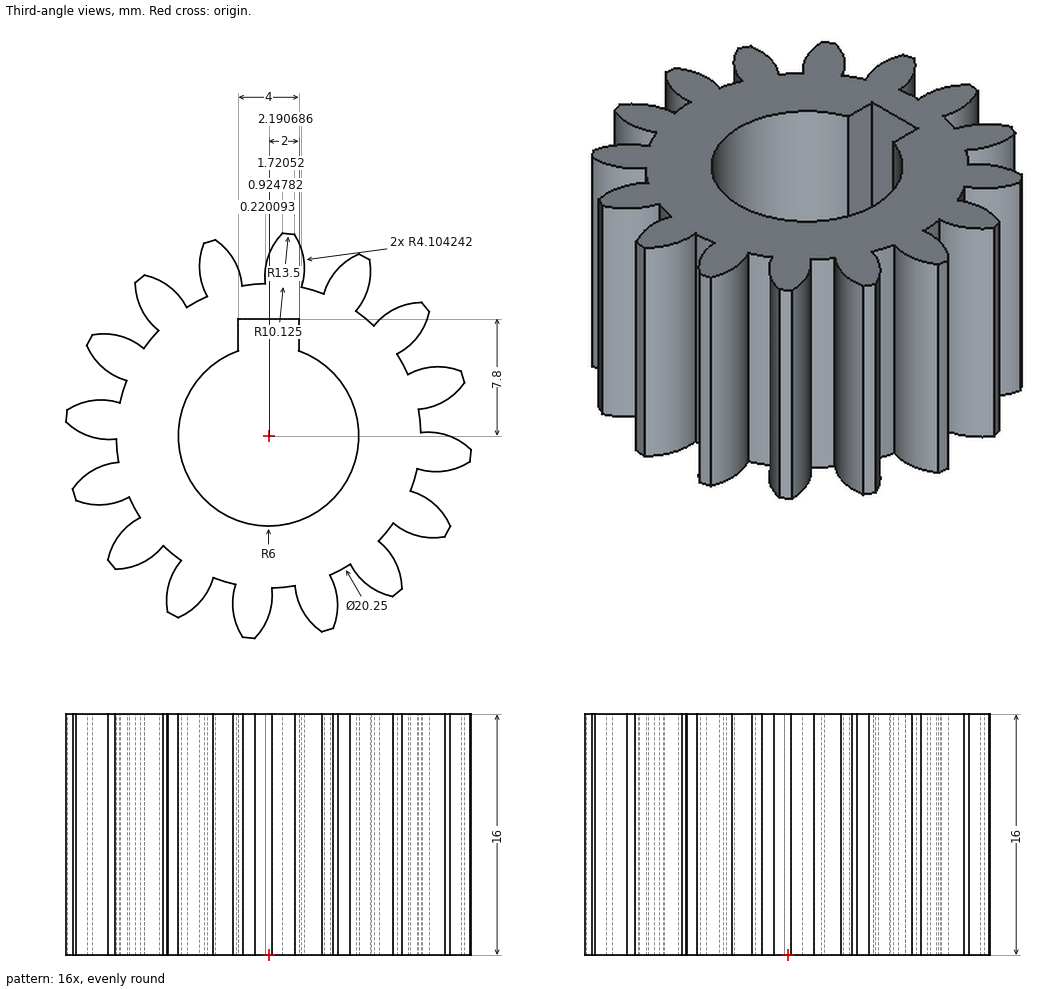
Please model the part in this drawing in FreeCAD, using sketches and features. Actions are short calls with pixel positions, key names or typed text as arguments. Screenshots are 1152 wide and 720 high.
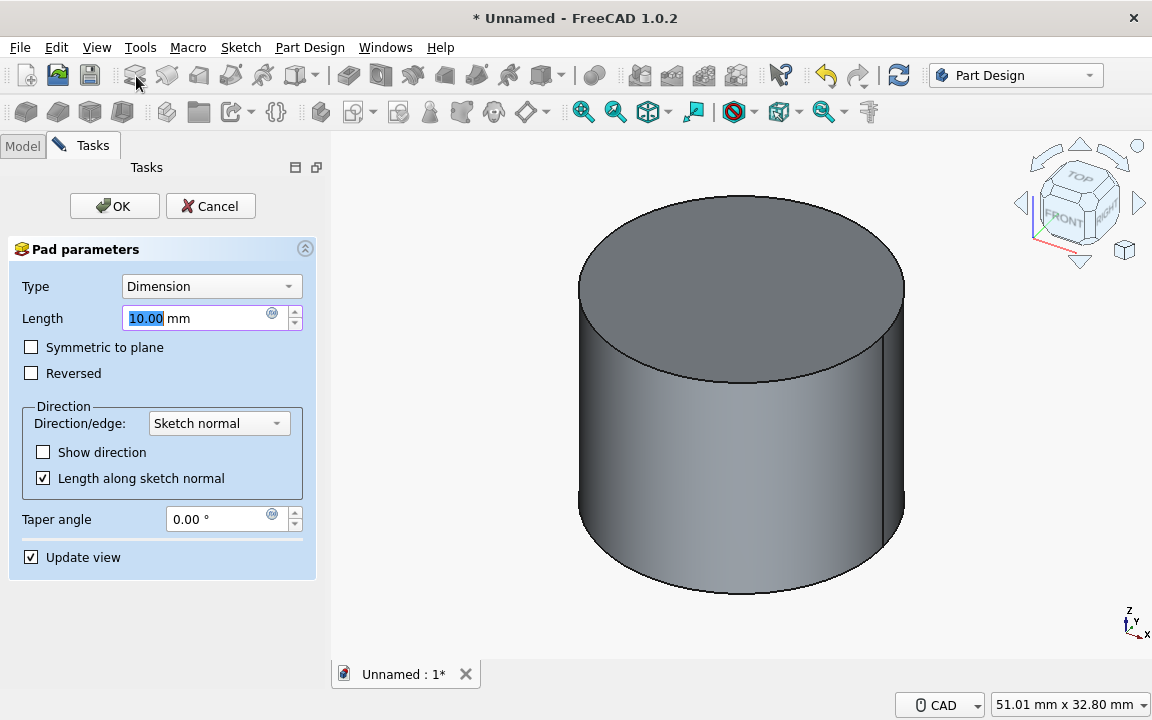
text(16)
key(Tab)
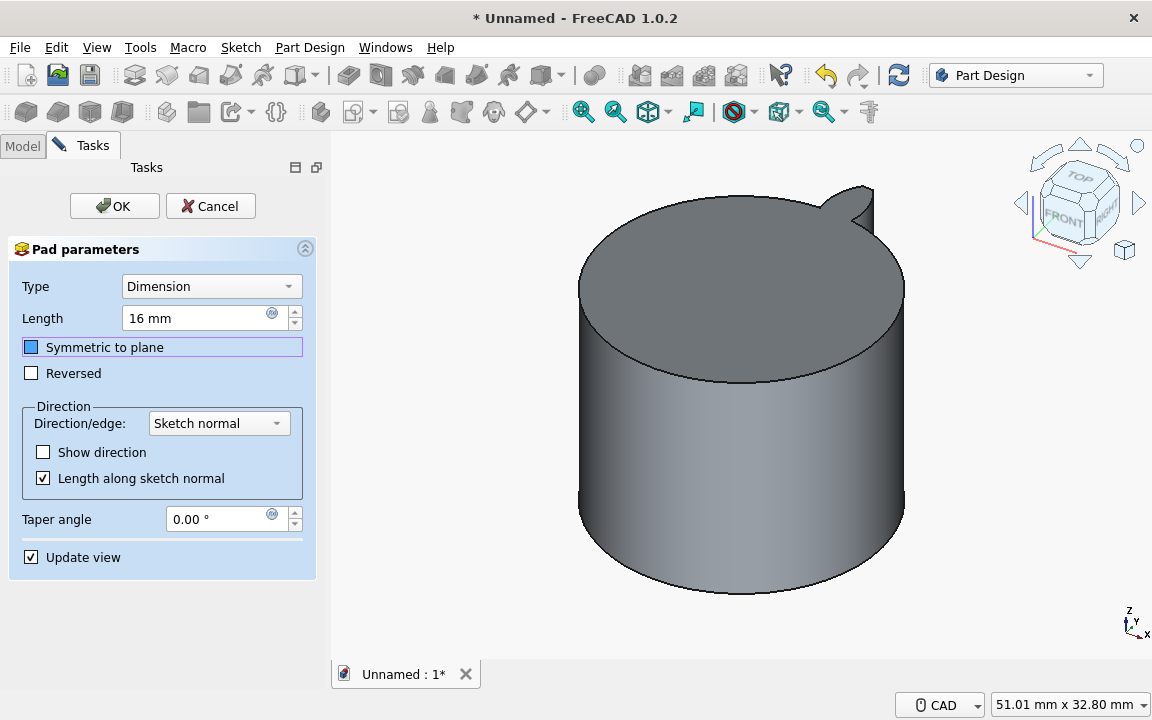
click(115, 206)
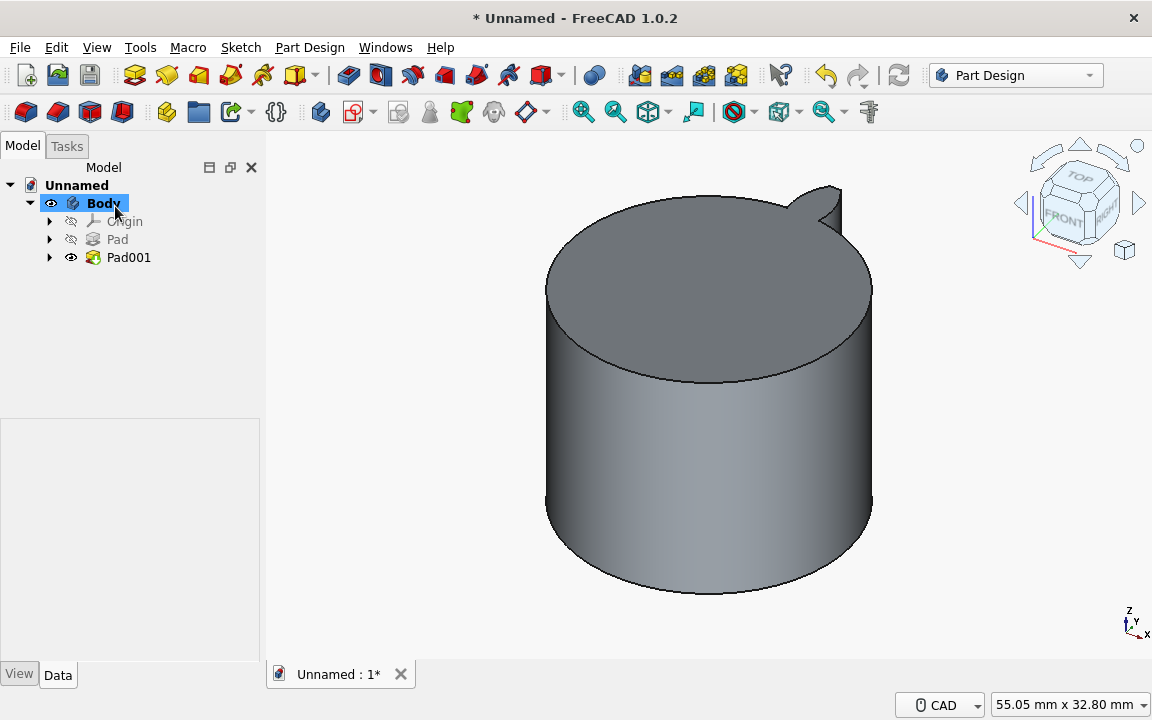
click(116, 257)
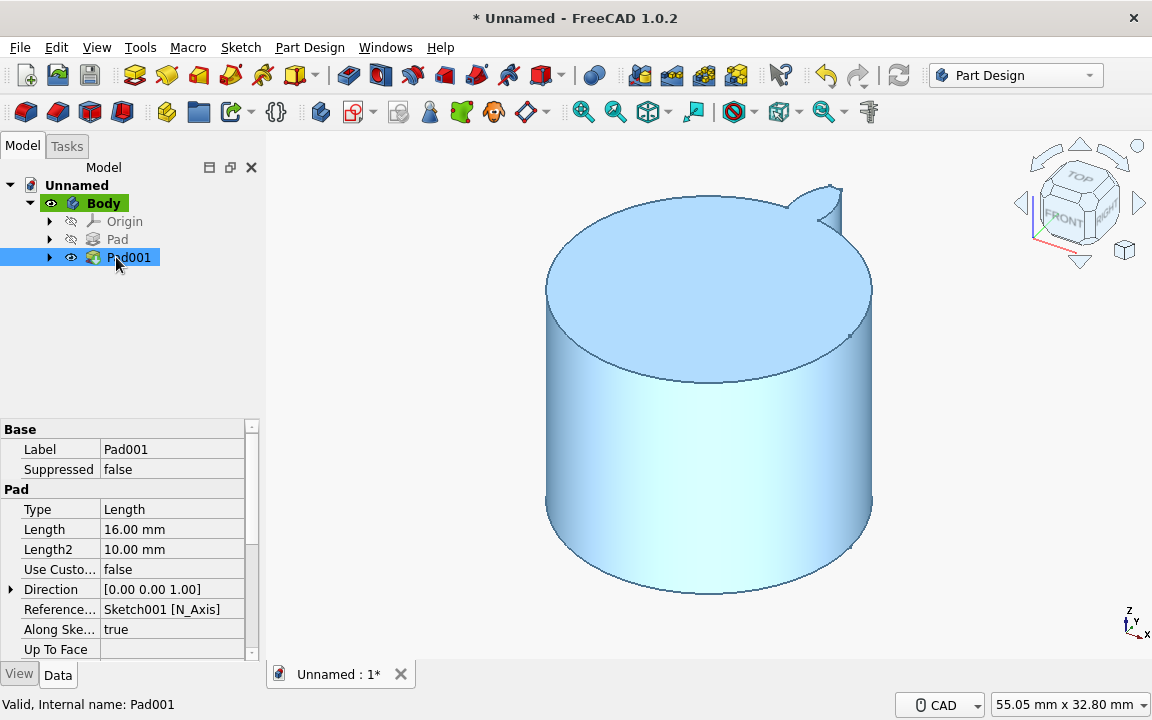
click(704, 76)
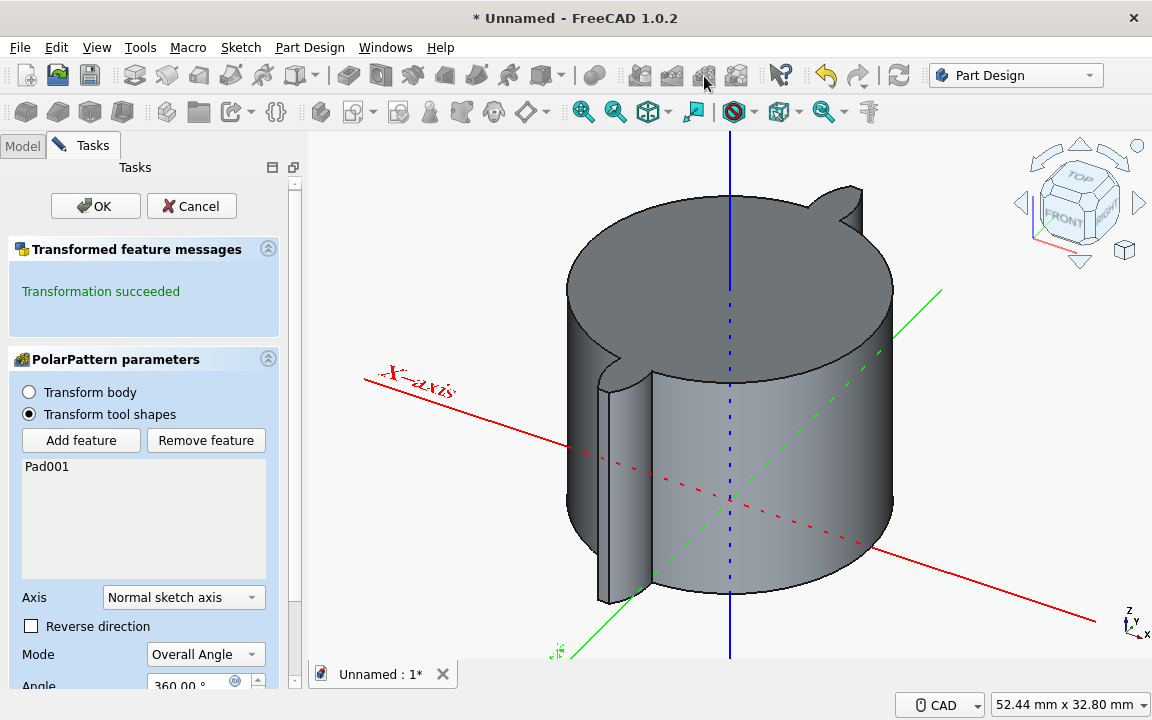
click(184, 598)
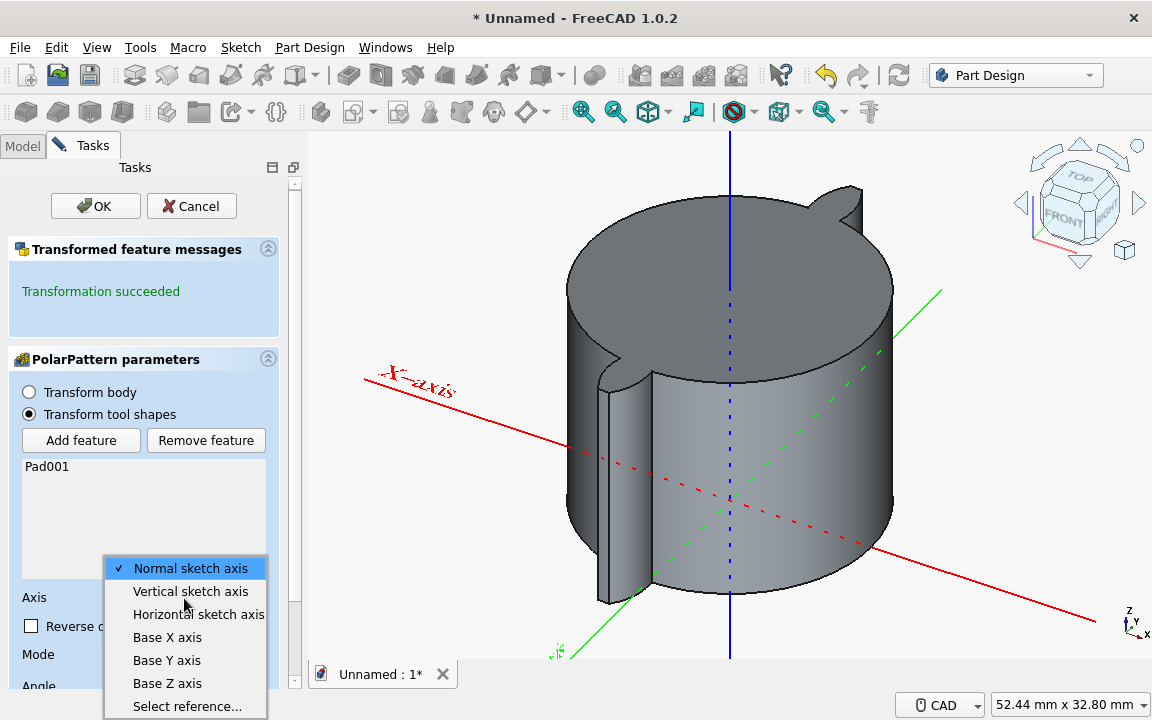
click(184, 684)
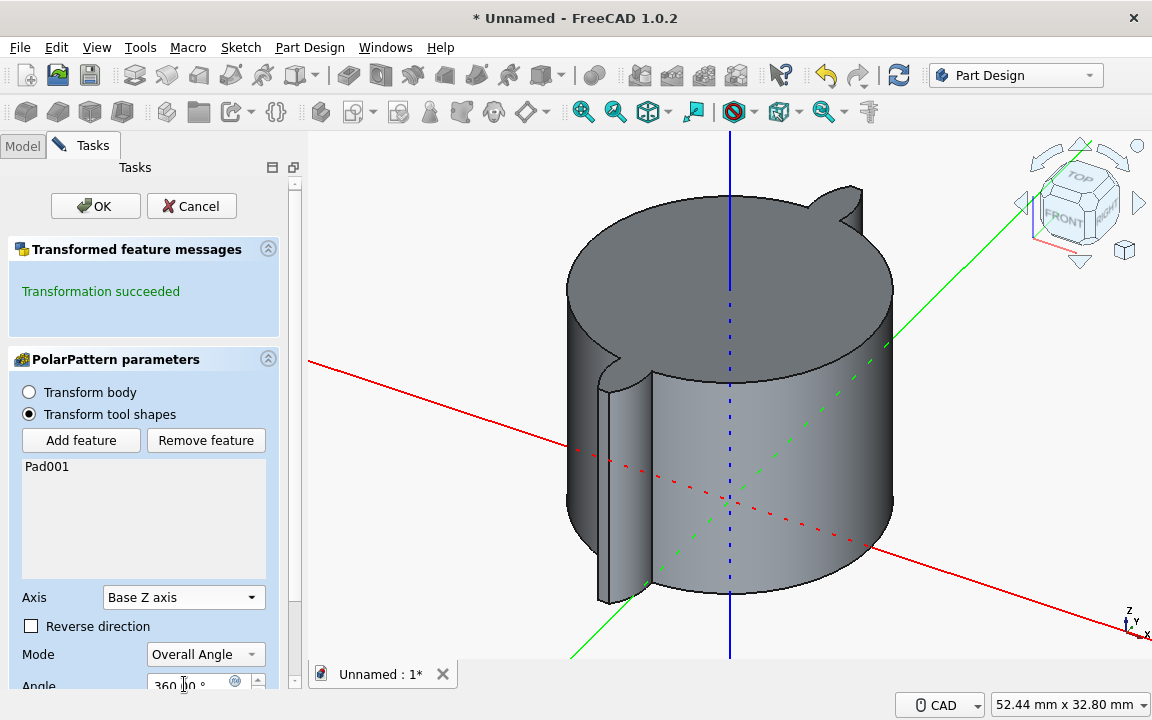
scroll(295, 432, down, 2)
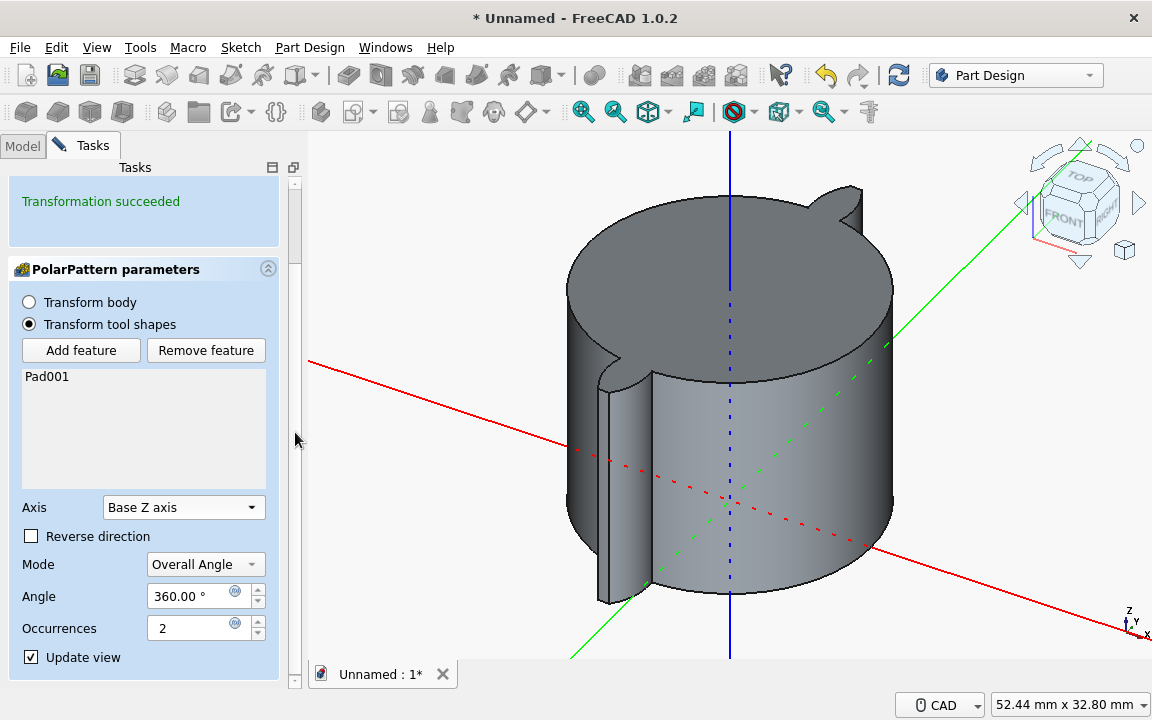
triple_click(198, 628)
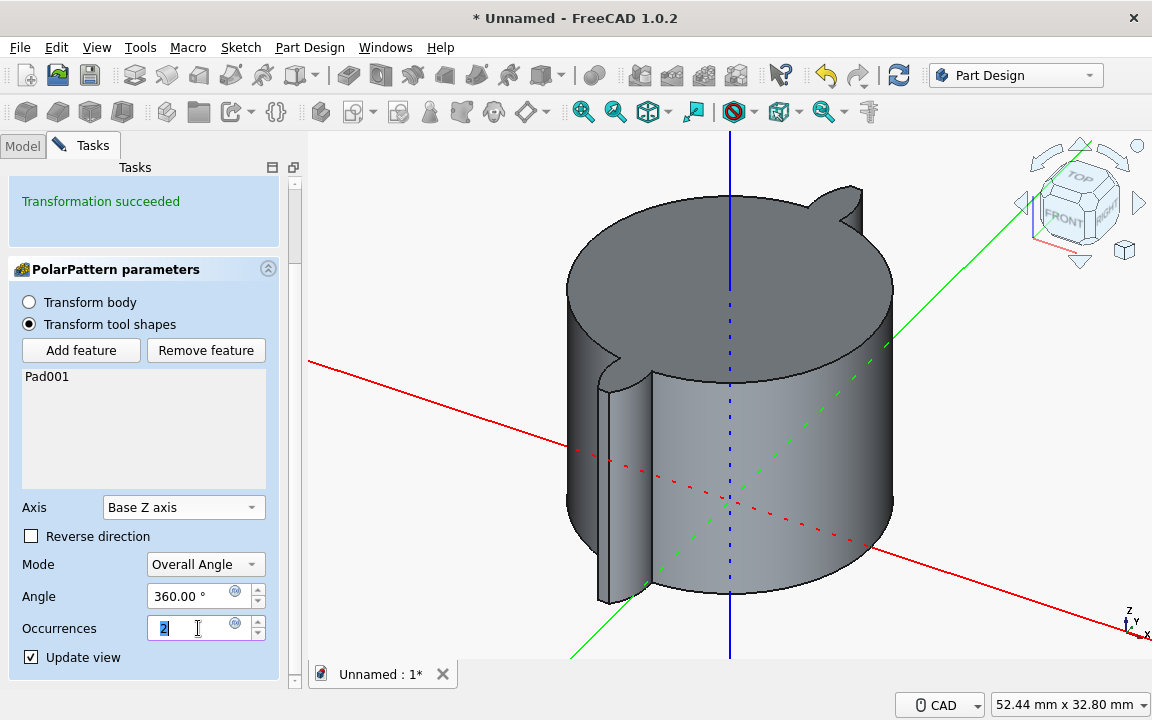
text(16)
key(Tab)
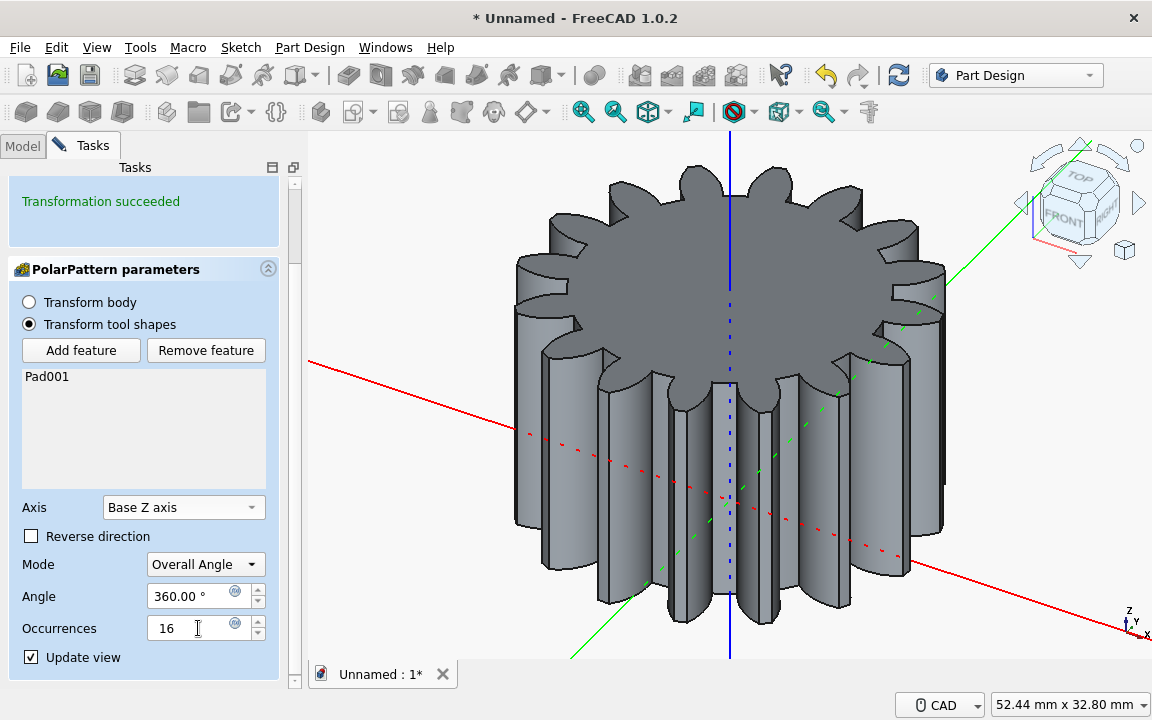
scroll(295, 432, up, 3)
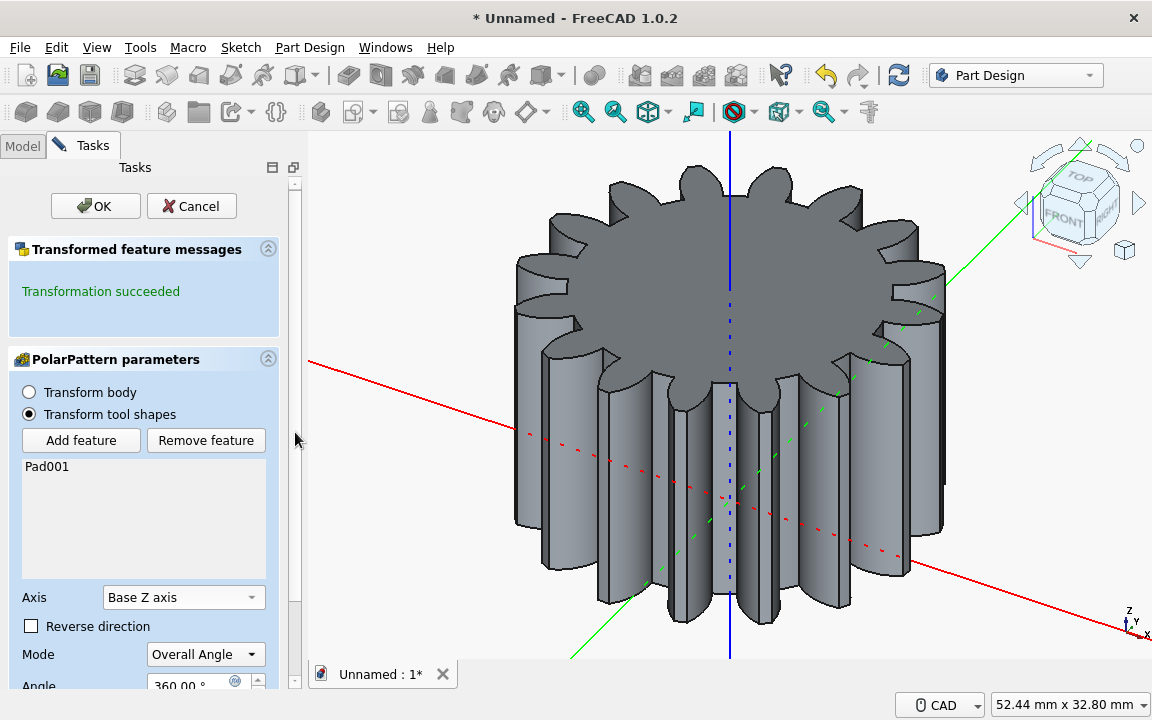
click(96, 206)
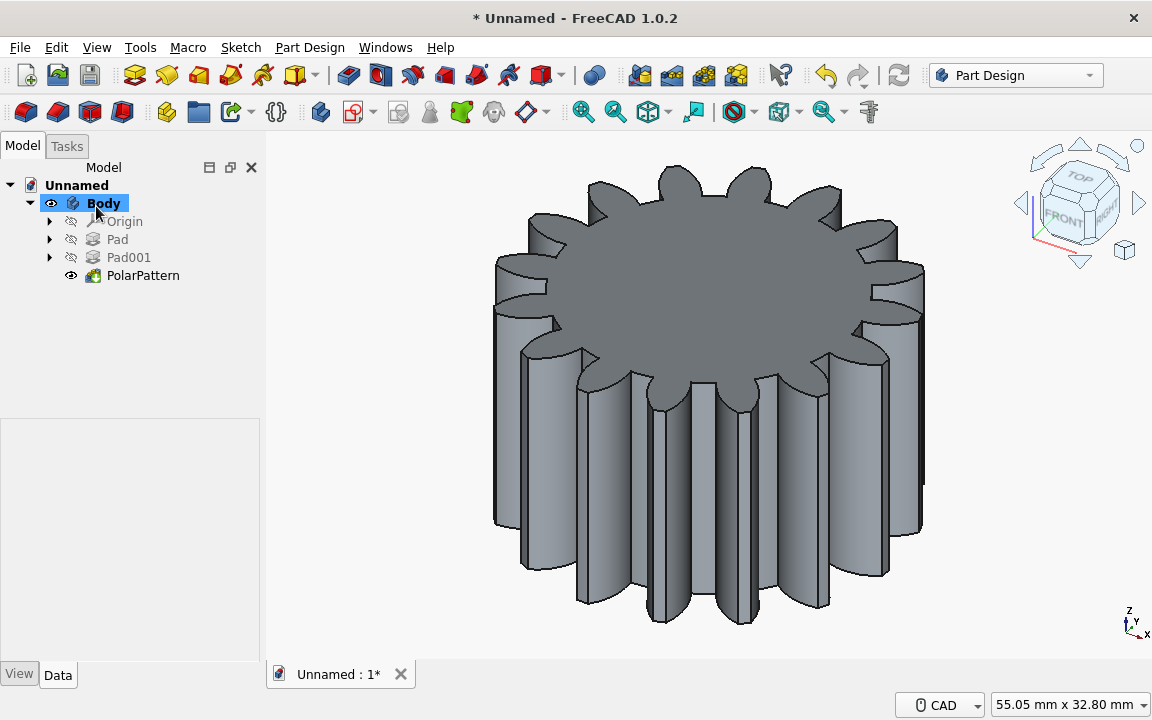
click(584, 112)